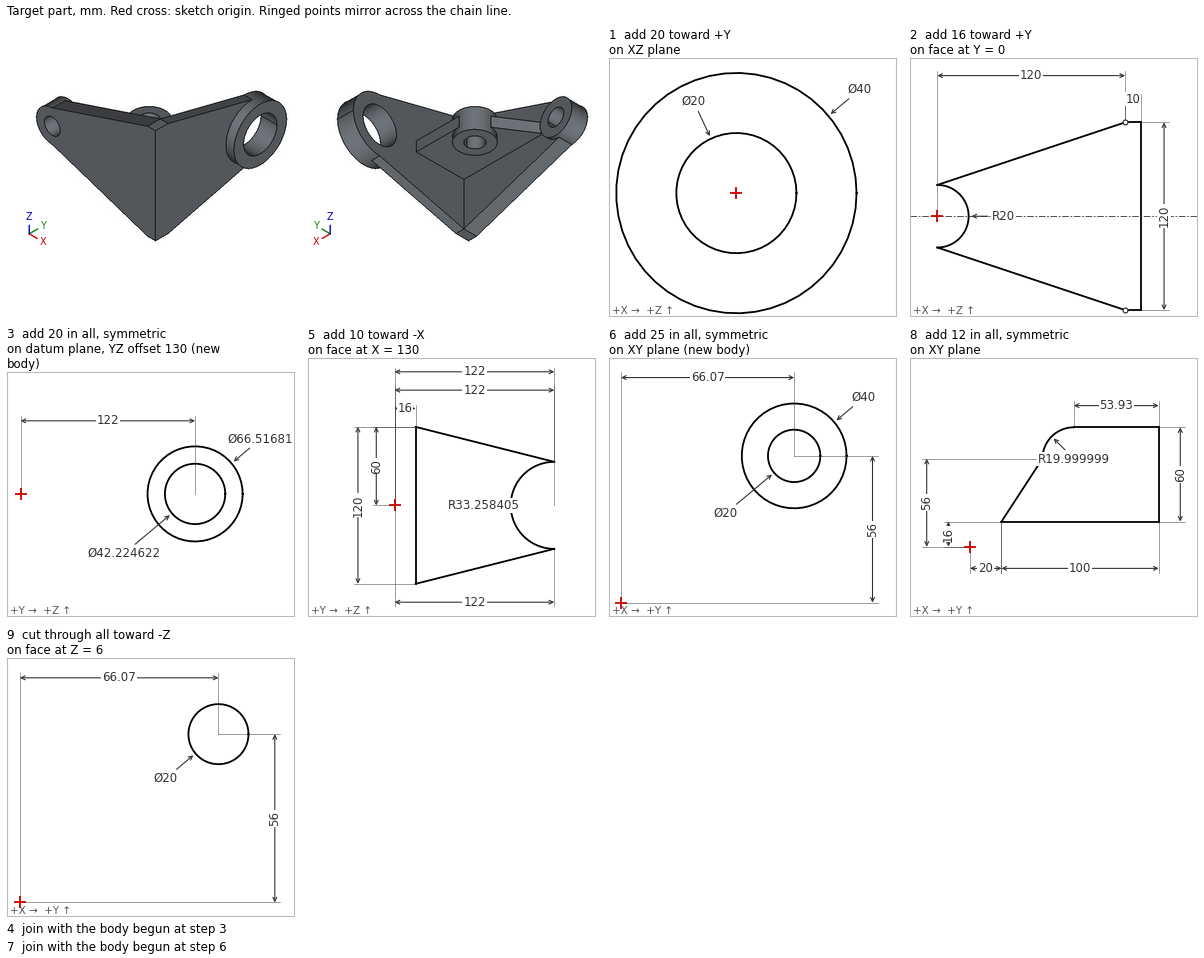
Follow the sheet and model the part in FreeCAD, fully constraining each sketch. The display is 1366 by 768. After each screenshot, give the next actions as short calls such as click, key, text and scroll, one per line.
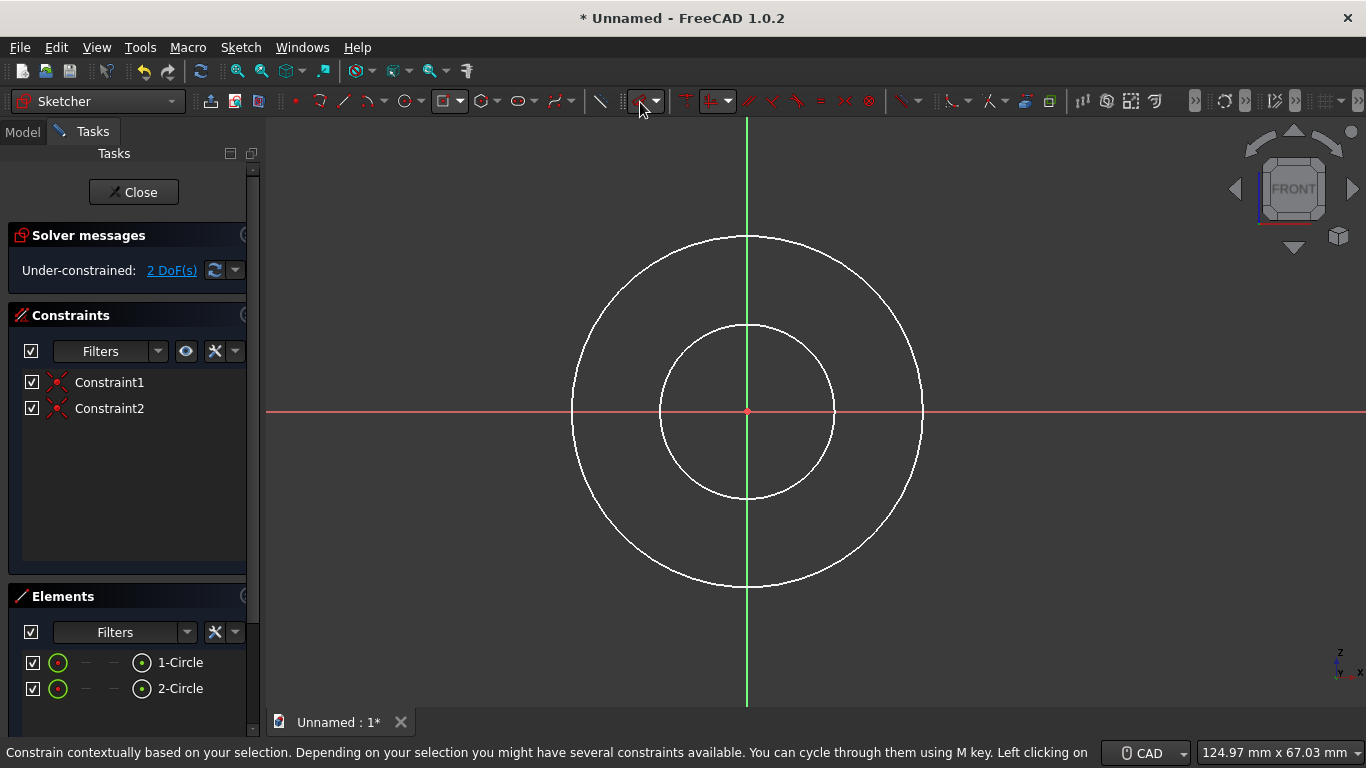
click(871, 287)
click(894, 264)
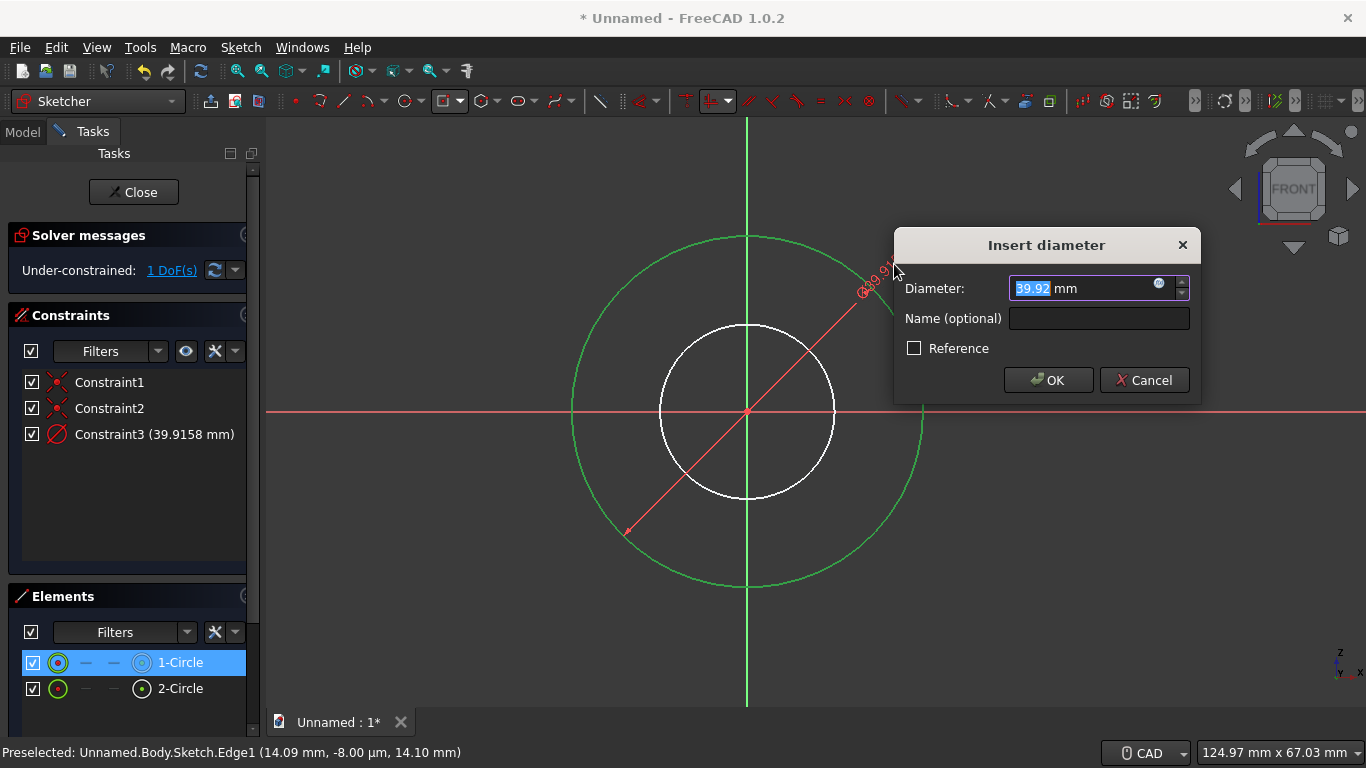
text(40)
key(Return)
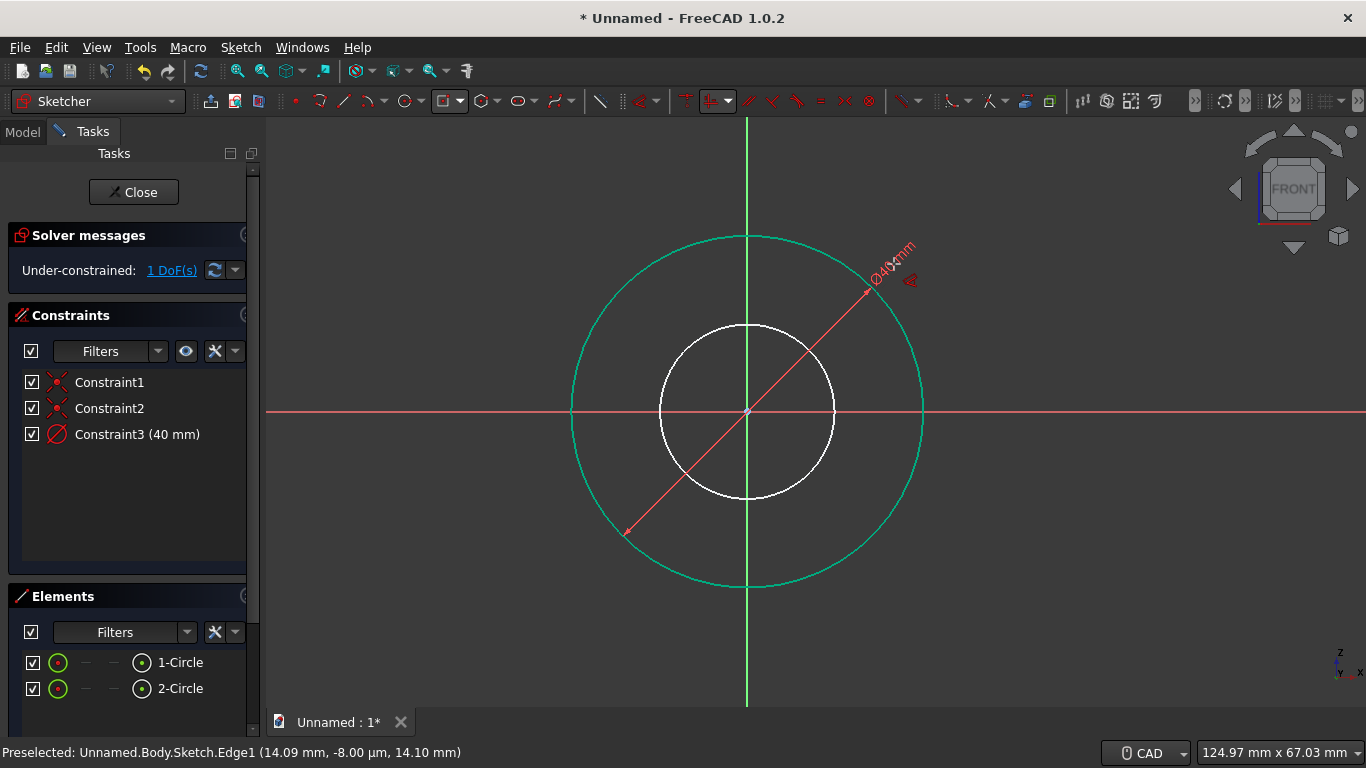
click(809, 350)
click(832, 327)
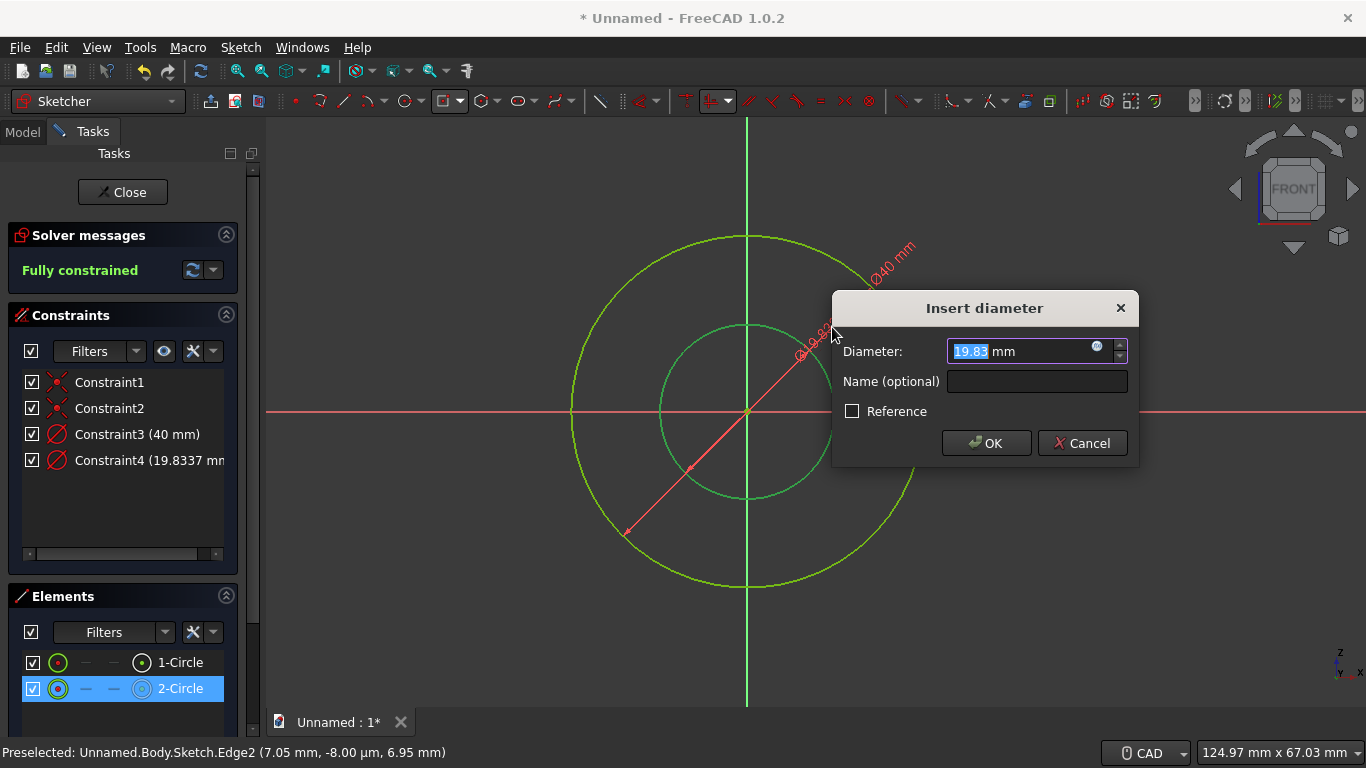
text(20)
key(Return)
key(Escape)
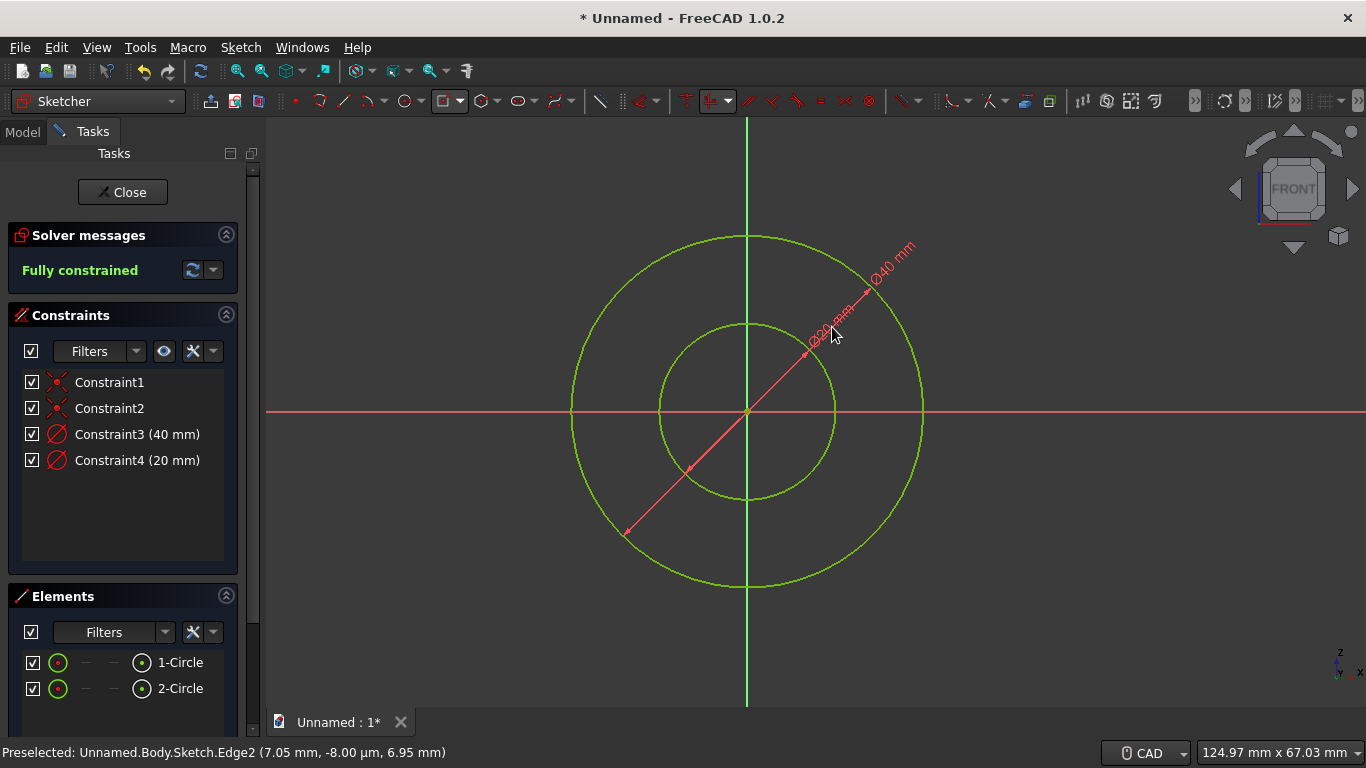
click(123, 192)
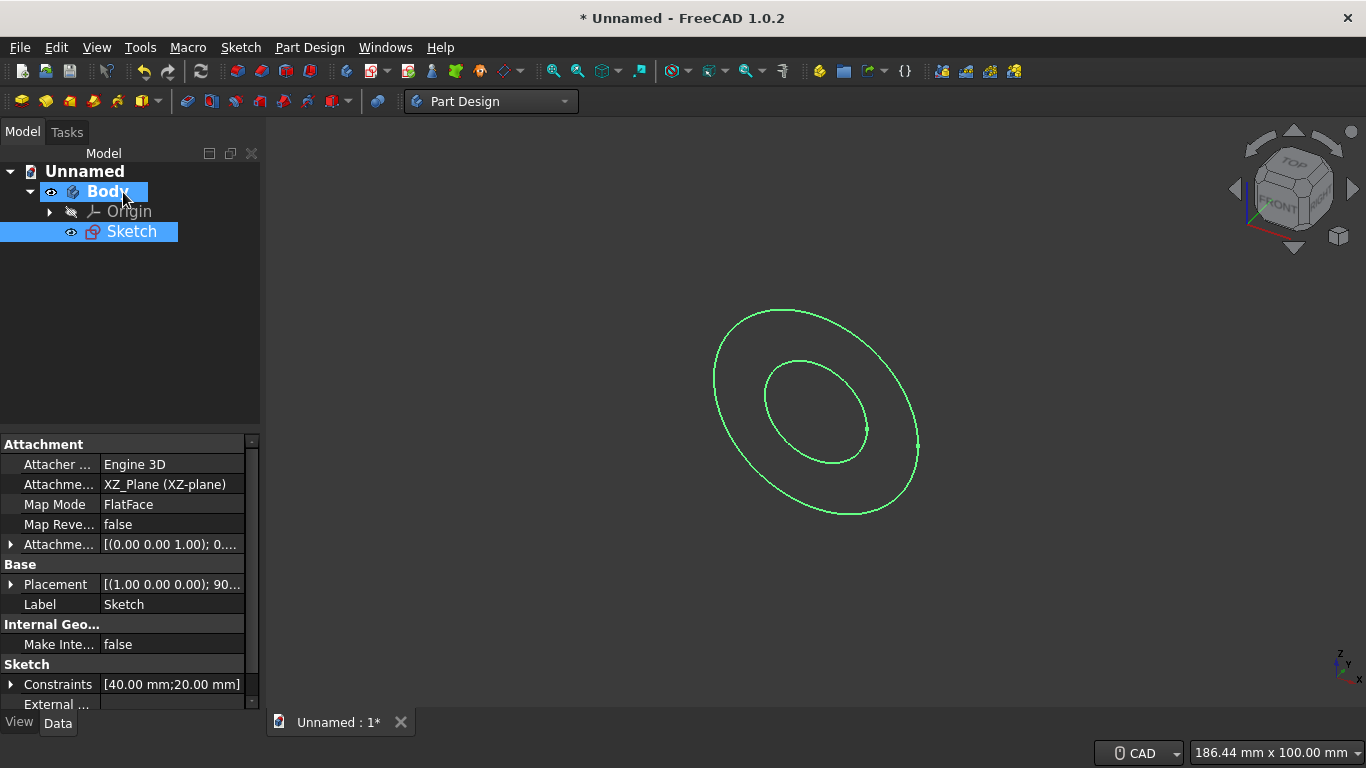
click(22, 102)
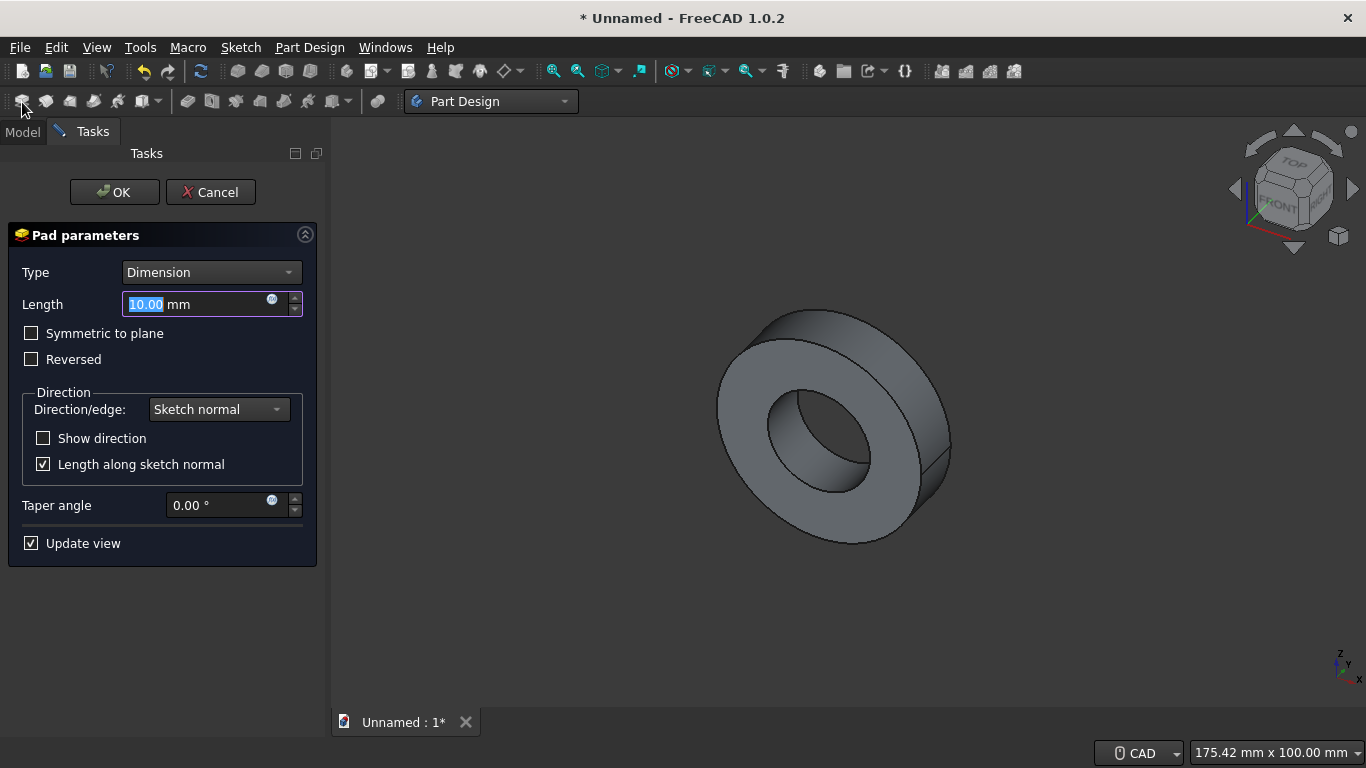
text(20)
key(Tab)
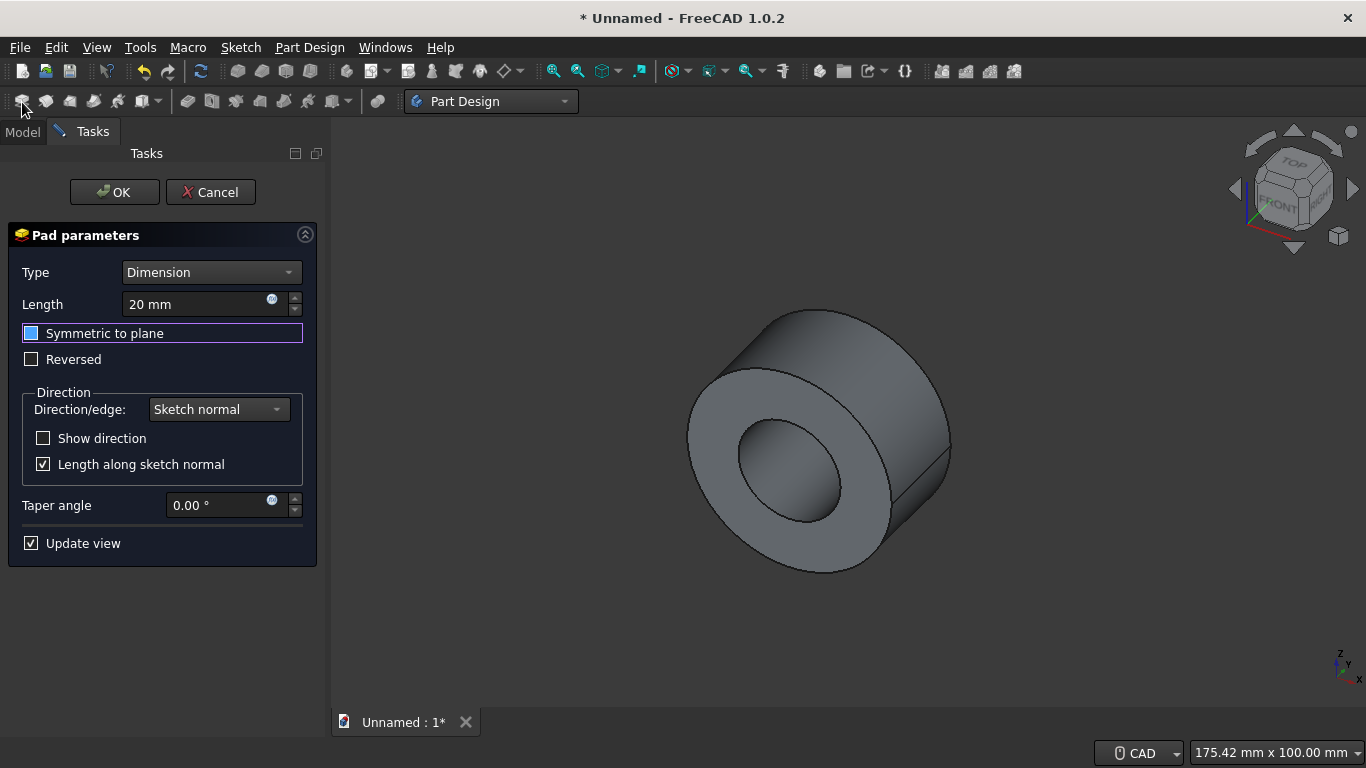
click(30, 359)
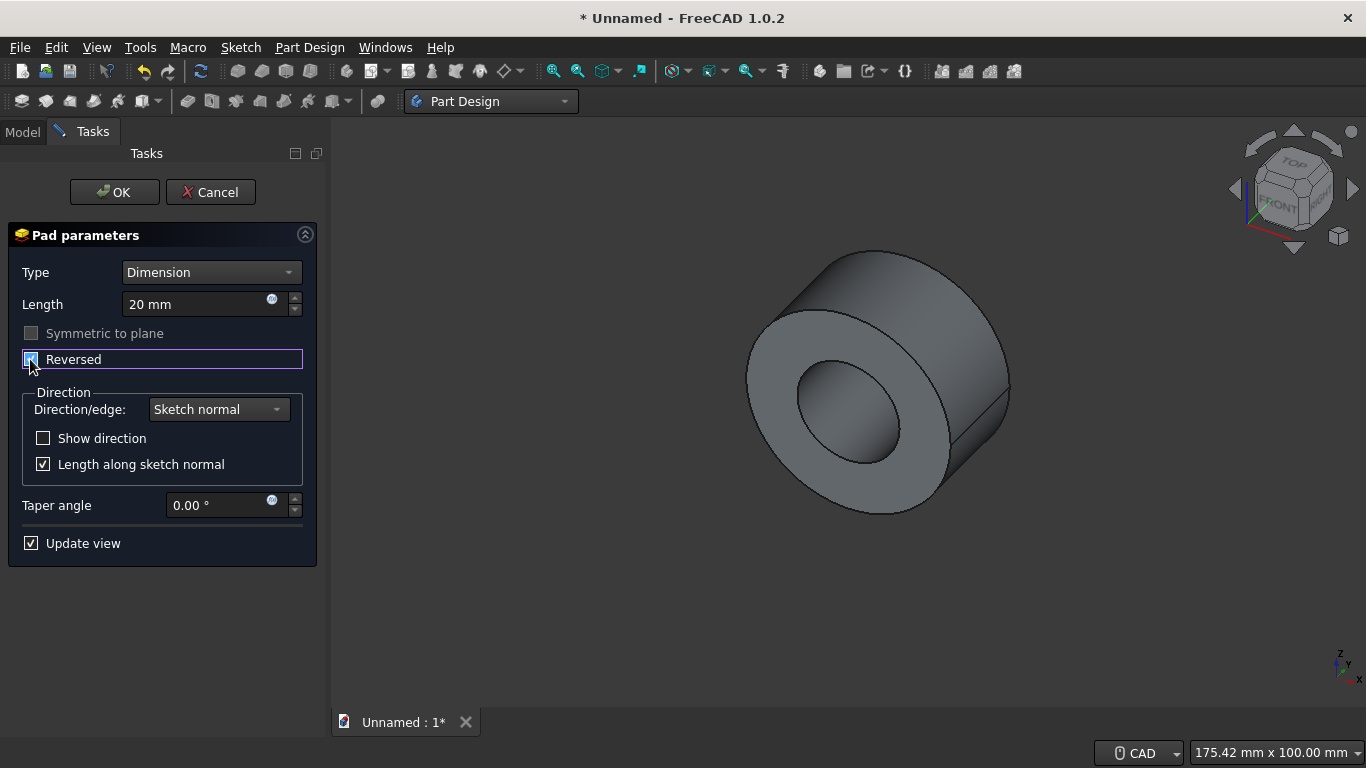
click(115, 192)